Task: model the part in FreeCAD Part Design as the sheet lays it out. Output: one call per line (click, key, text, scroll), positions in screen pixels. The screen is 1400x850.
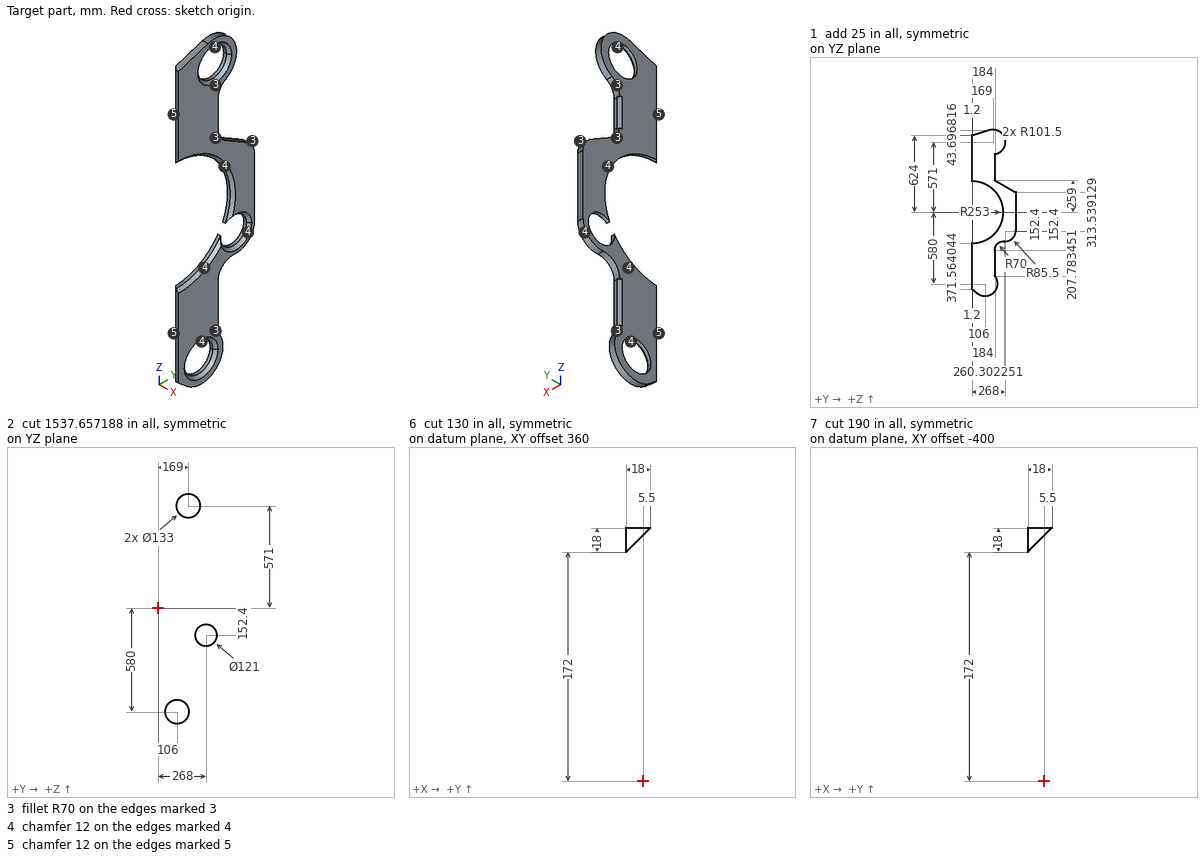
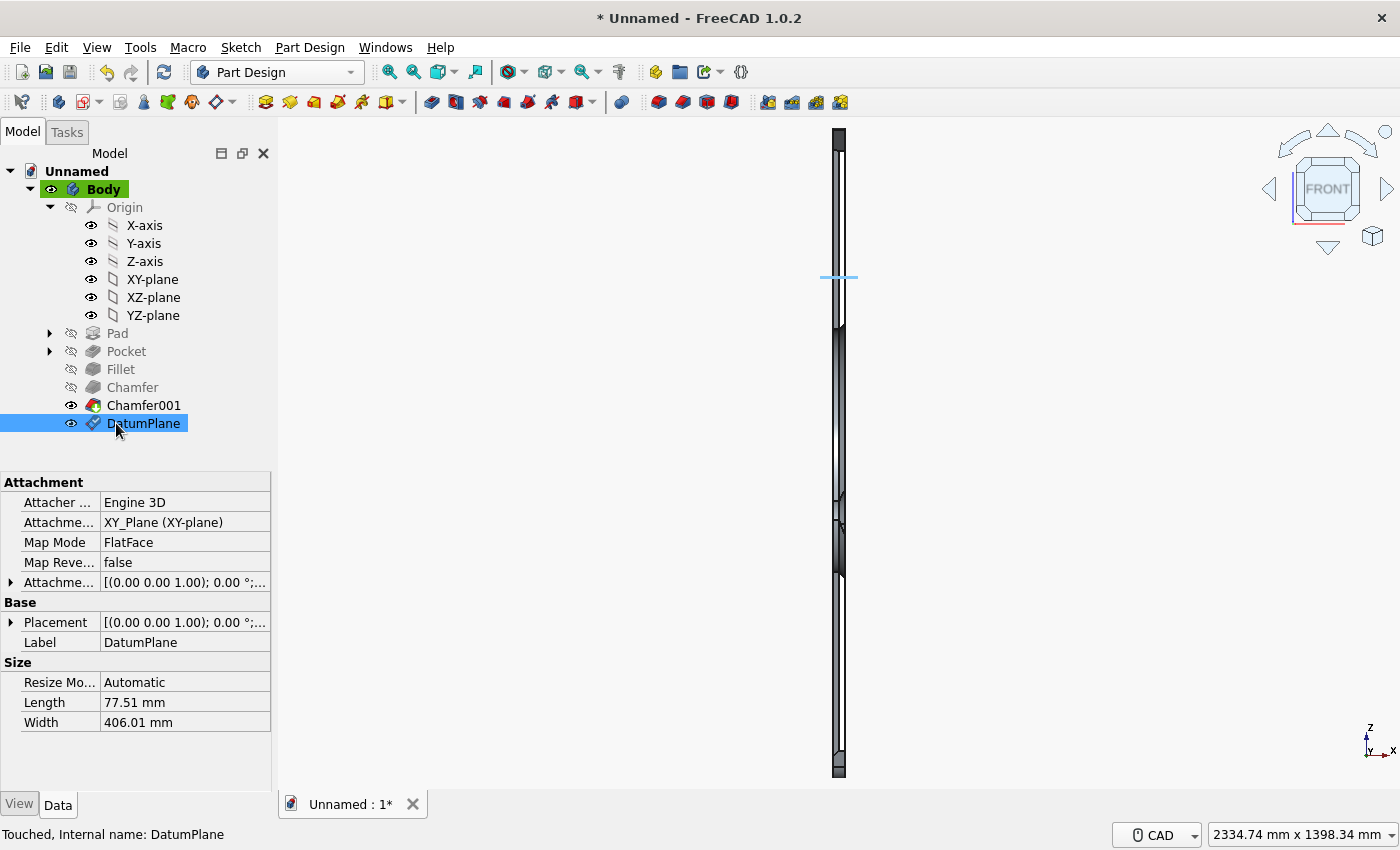
click(84, 102)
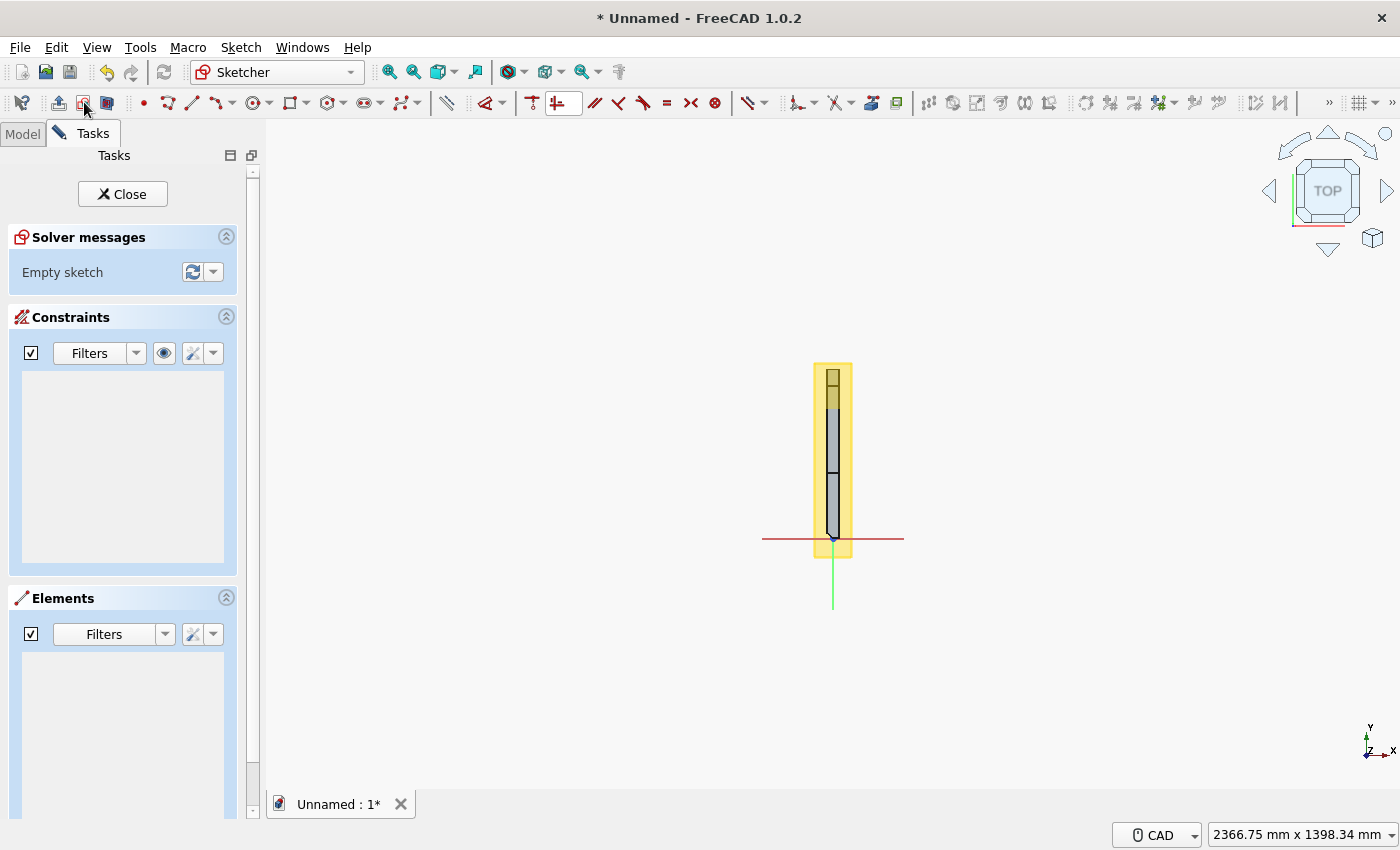
key(q)
key(s)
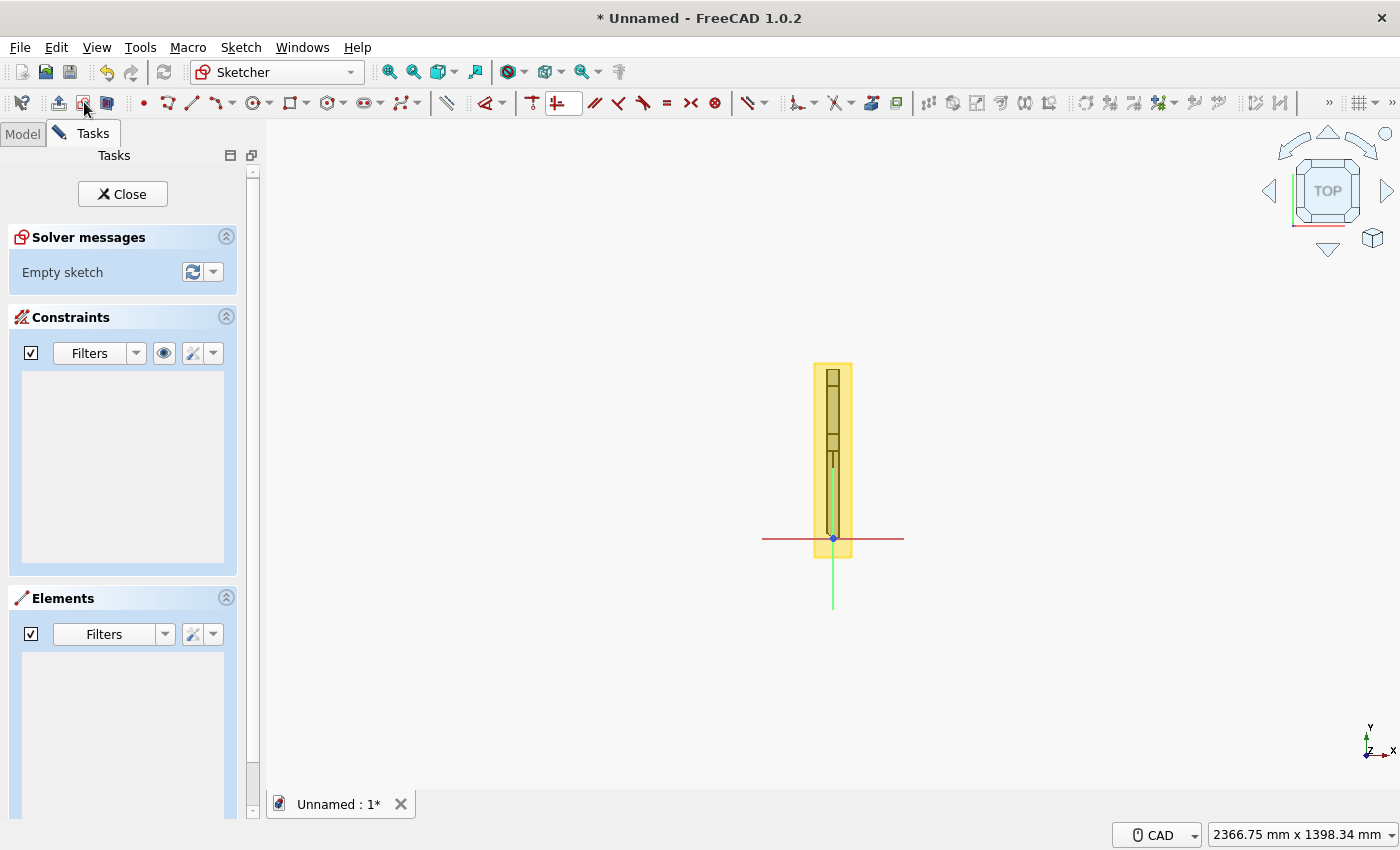
scroll(835, 452, up, 15)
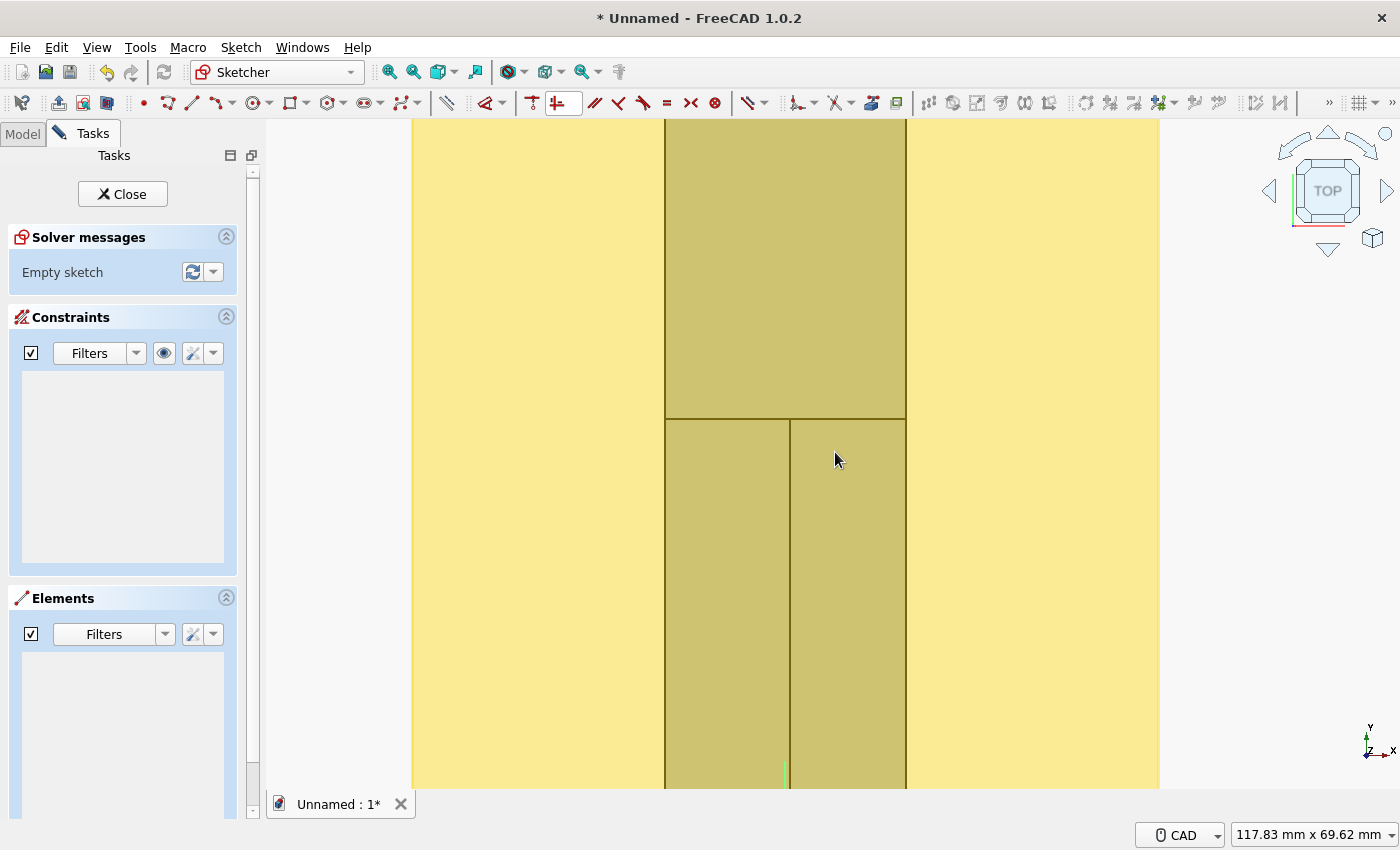
scroll(744, 444, up, 5)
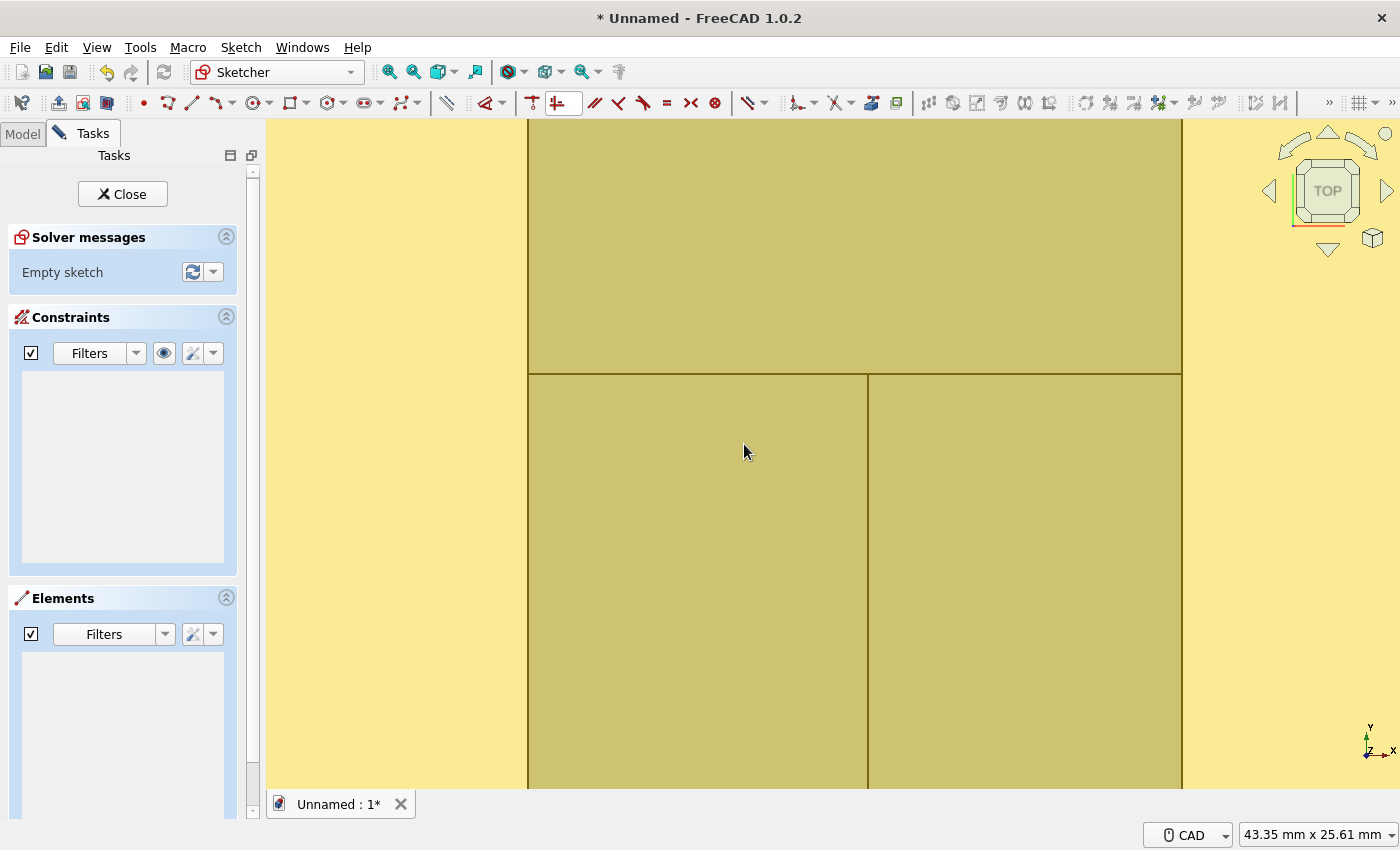
key(g)
key(m)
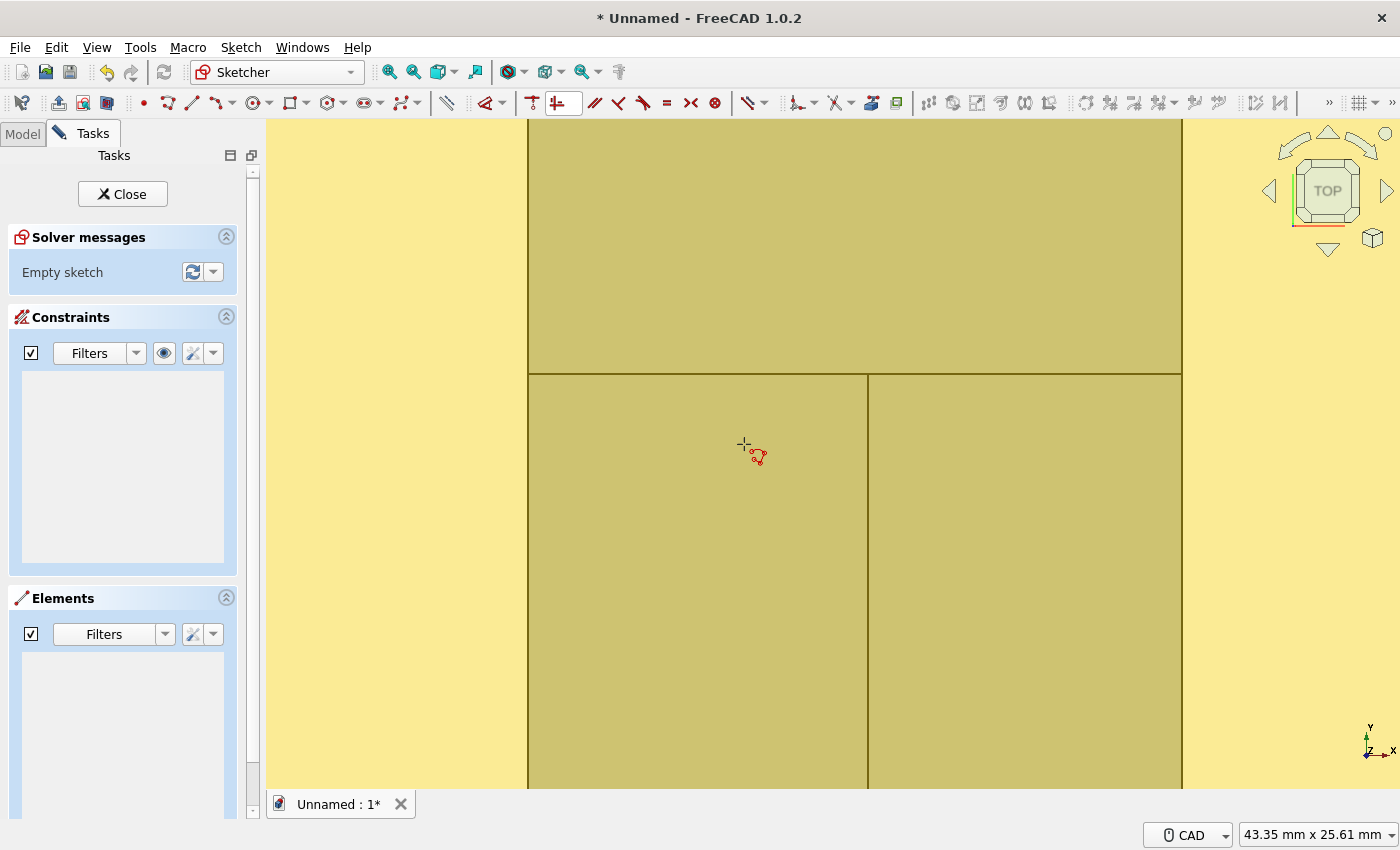
click(528, 688)
click(999, 217)
click(528, 217)
click(528, 689)
key(Escape)
key(Escape)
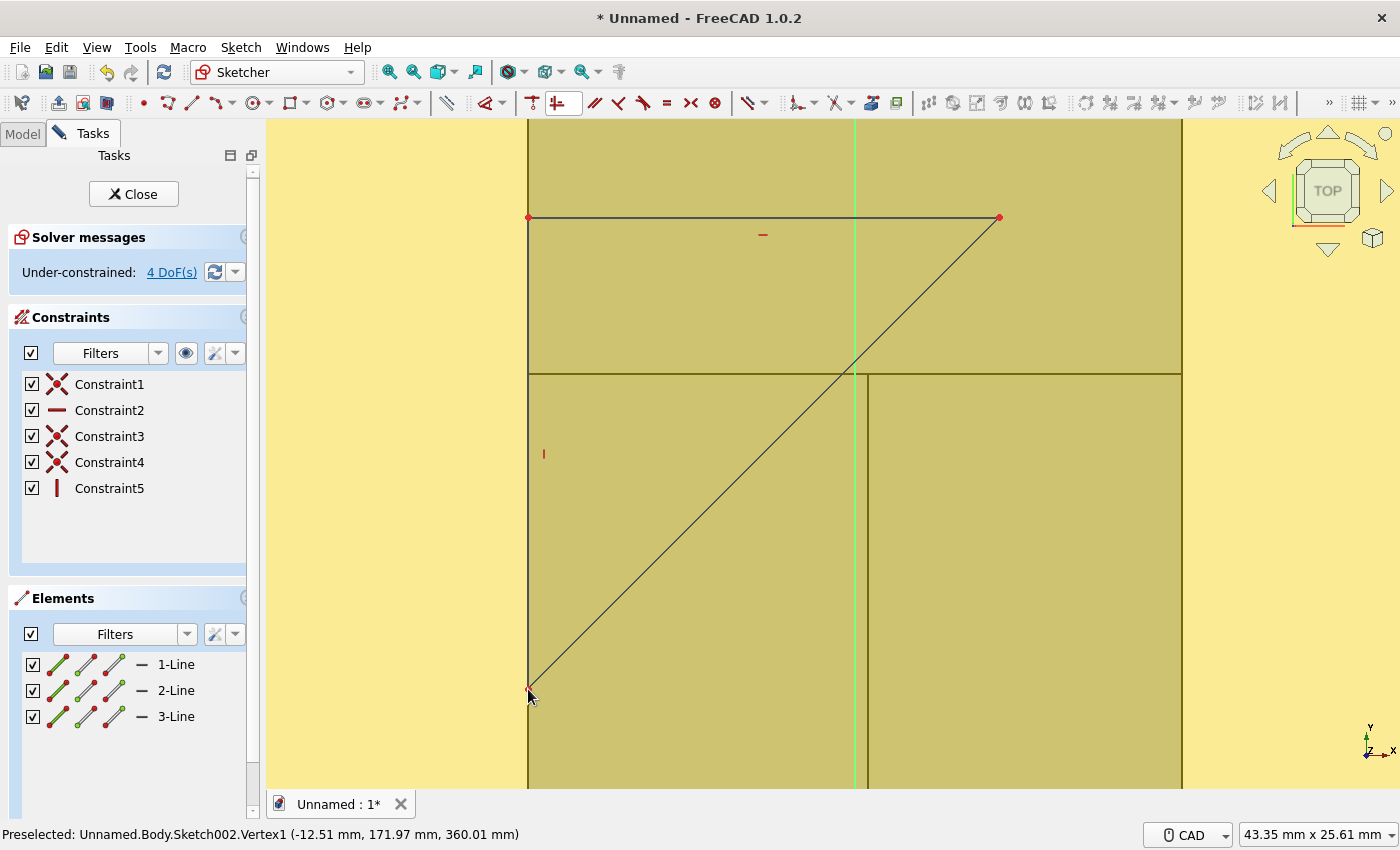
key(d)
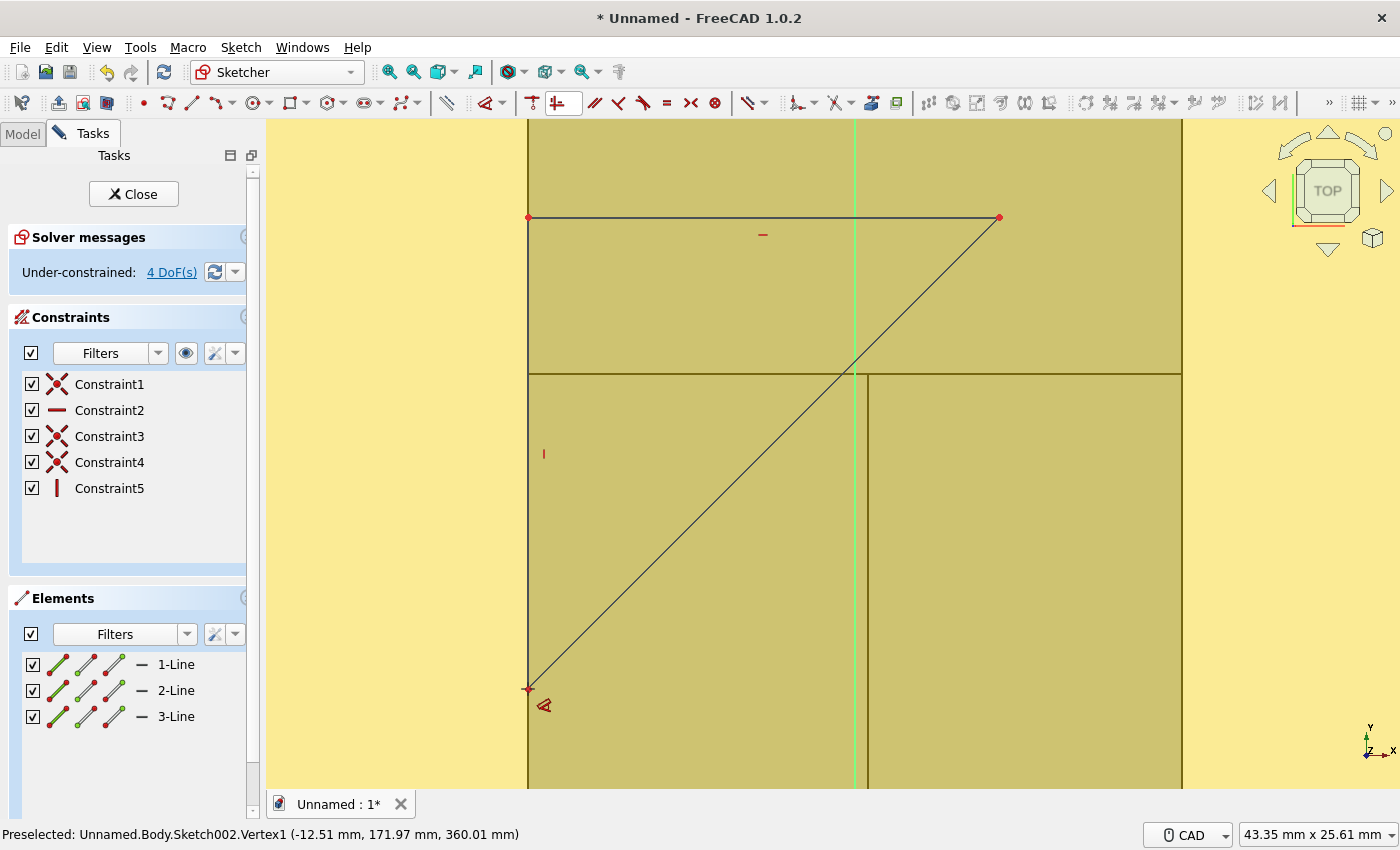
click(858, 218)
click(763, 184)